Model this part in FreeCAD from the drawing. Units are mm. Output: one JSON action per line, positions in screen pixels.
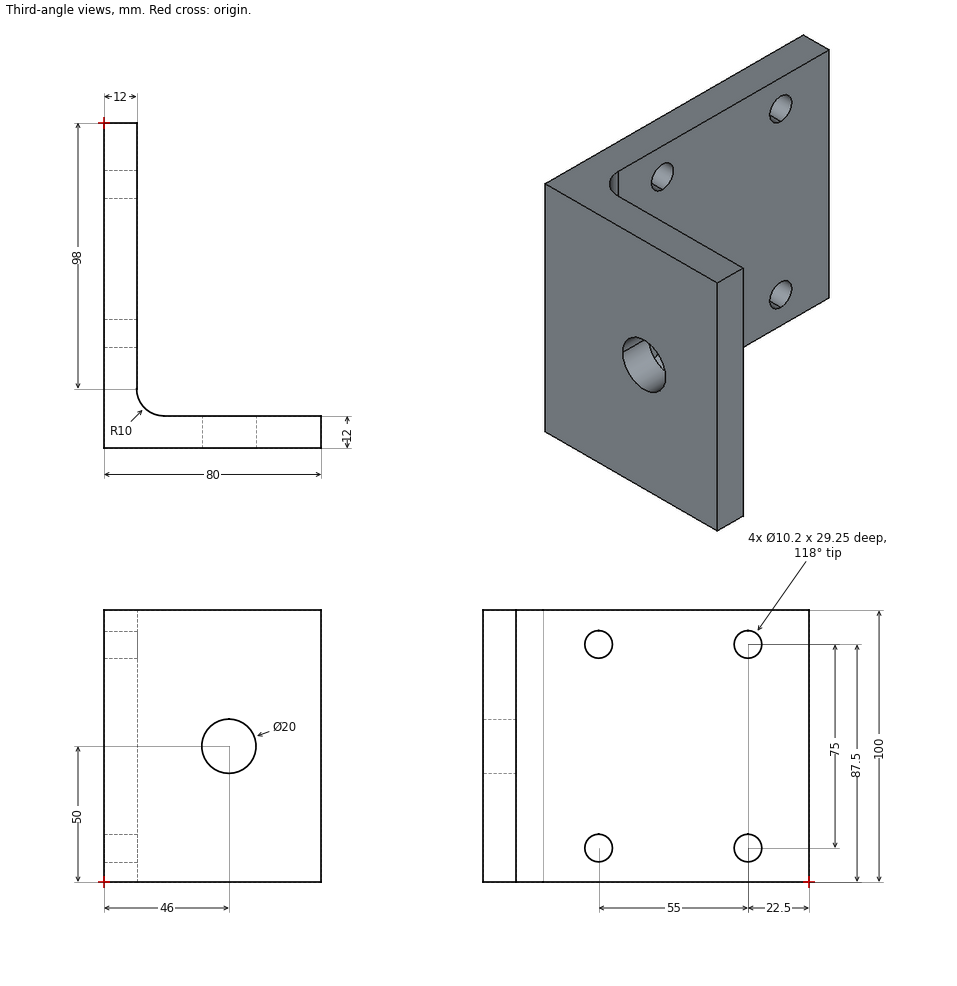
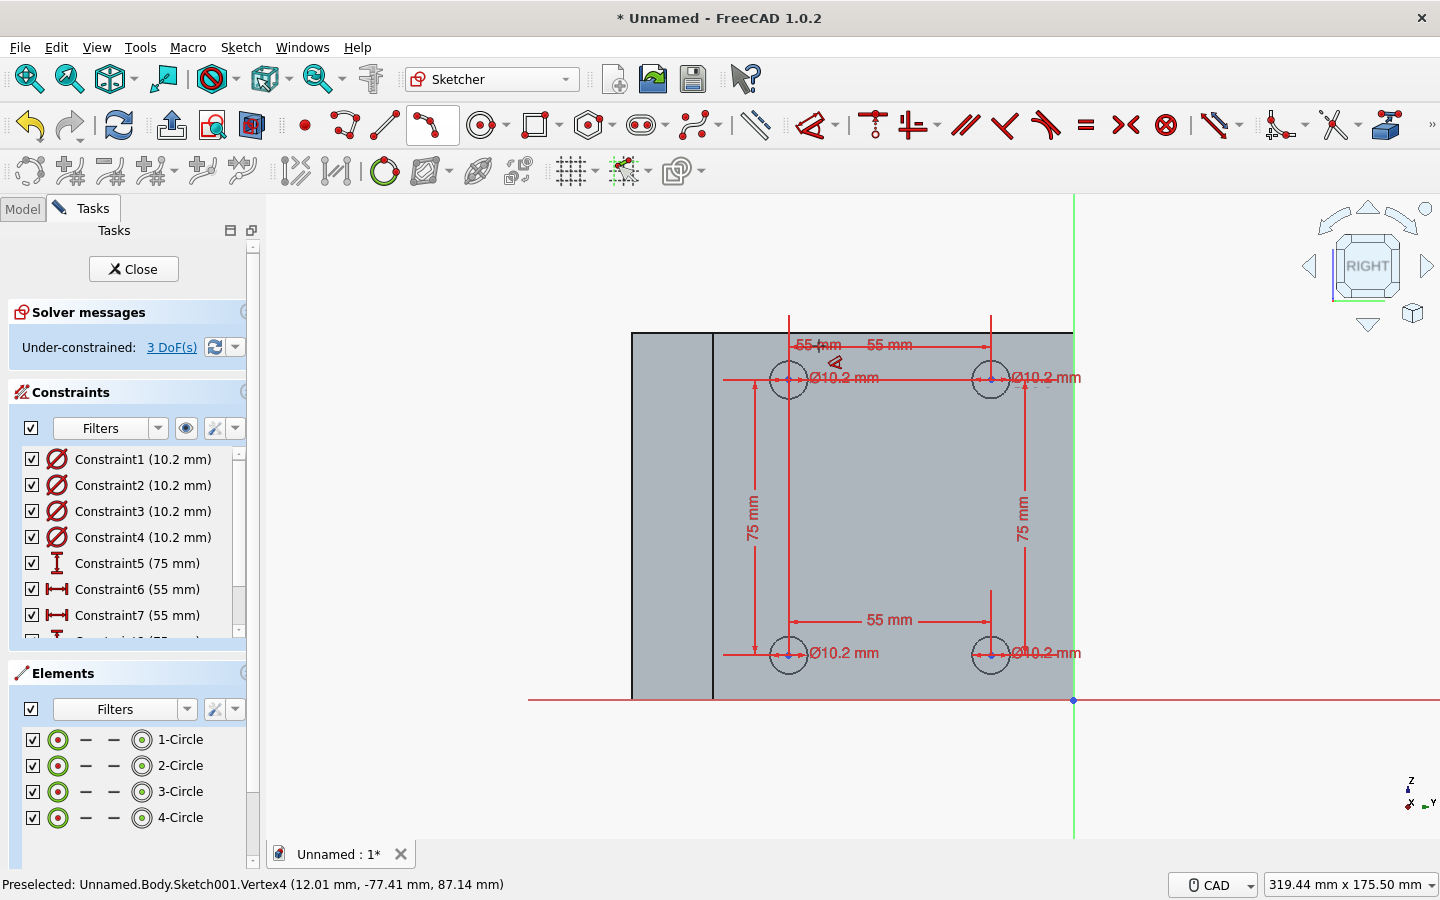
{"action": "left_click", "coordinate": [789, 655]}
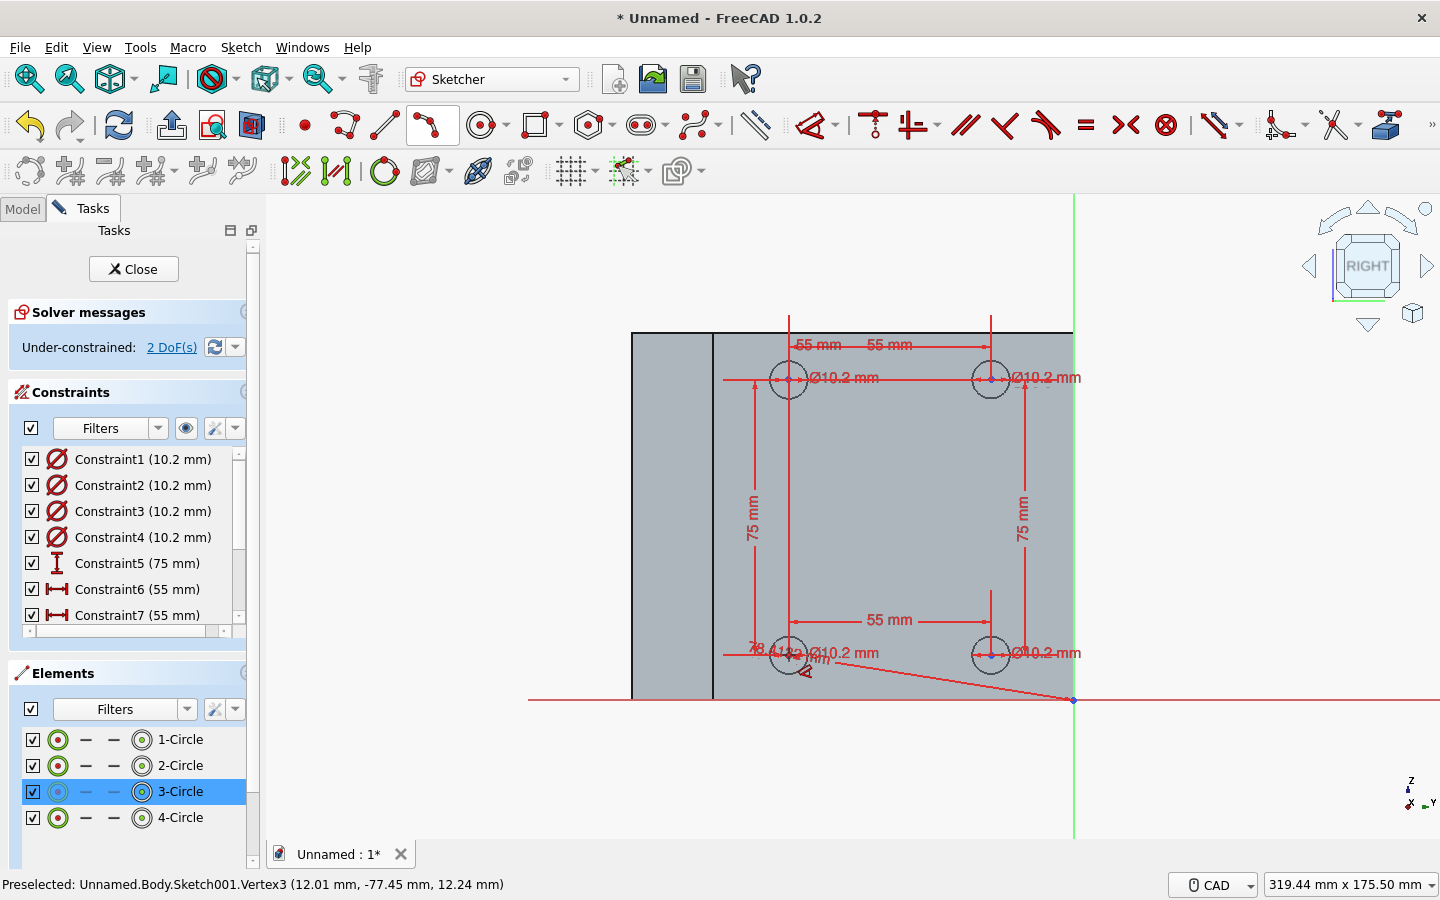
{"action": "left_click", "coordinate": [789, 380]}
{"action": "left_click", "coordinate": [755, 454]}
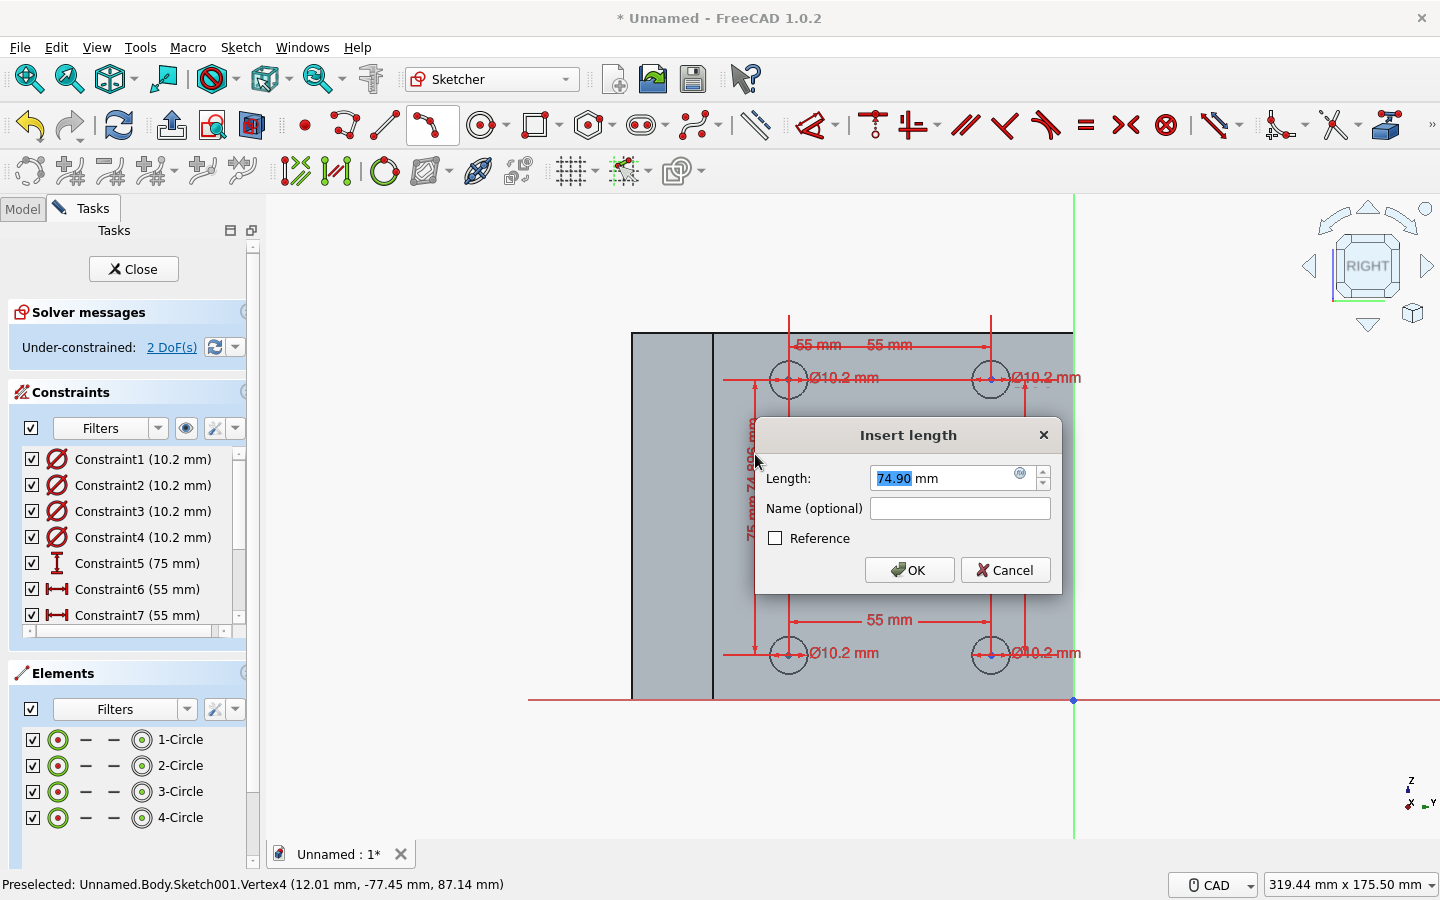
{"action": "type", "text": "75"}
{"action": "key", "text": "Return"}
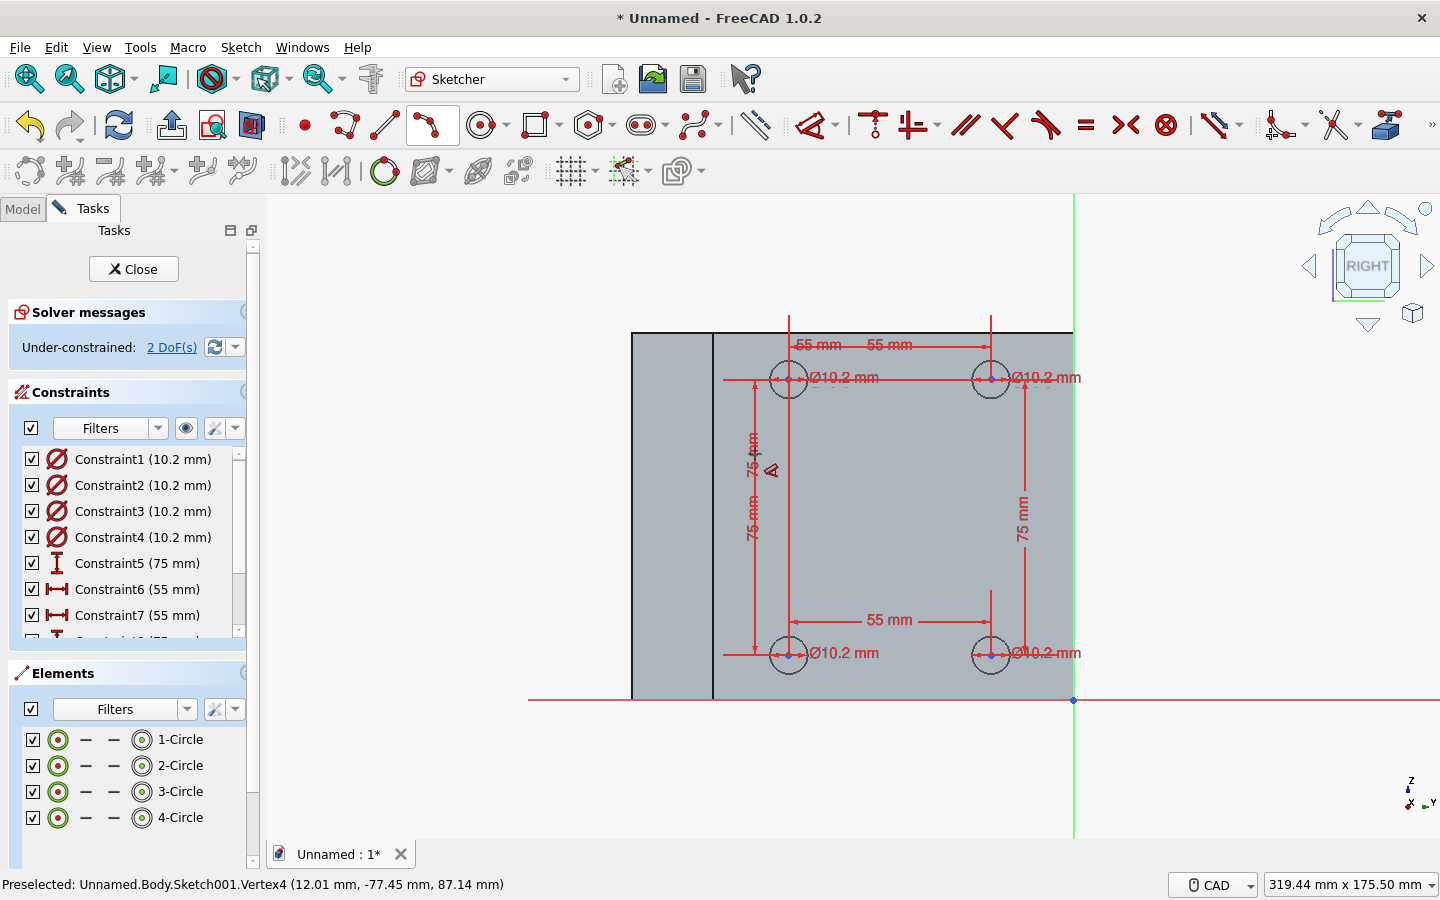
{"action": "left_click", "coordinate": [991, 380]}
{"action": "left_click", "coordinate": [1032, 734]}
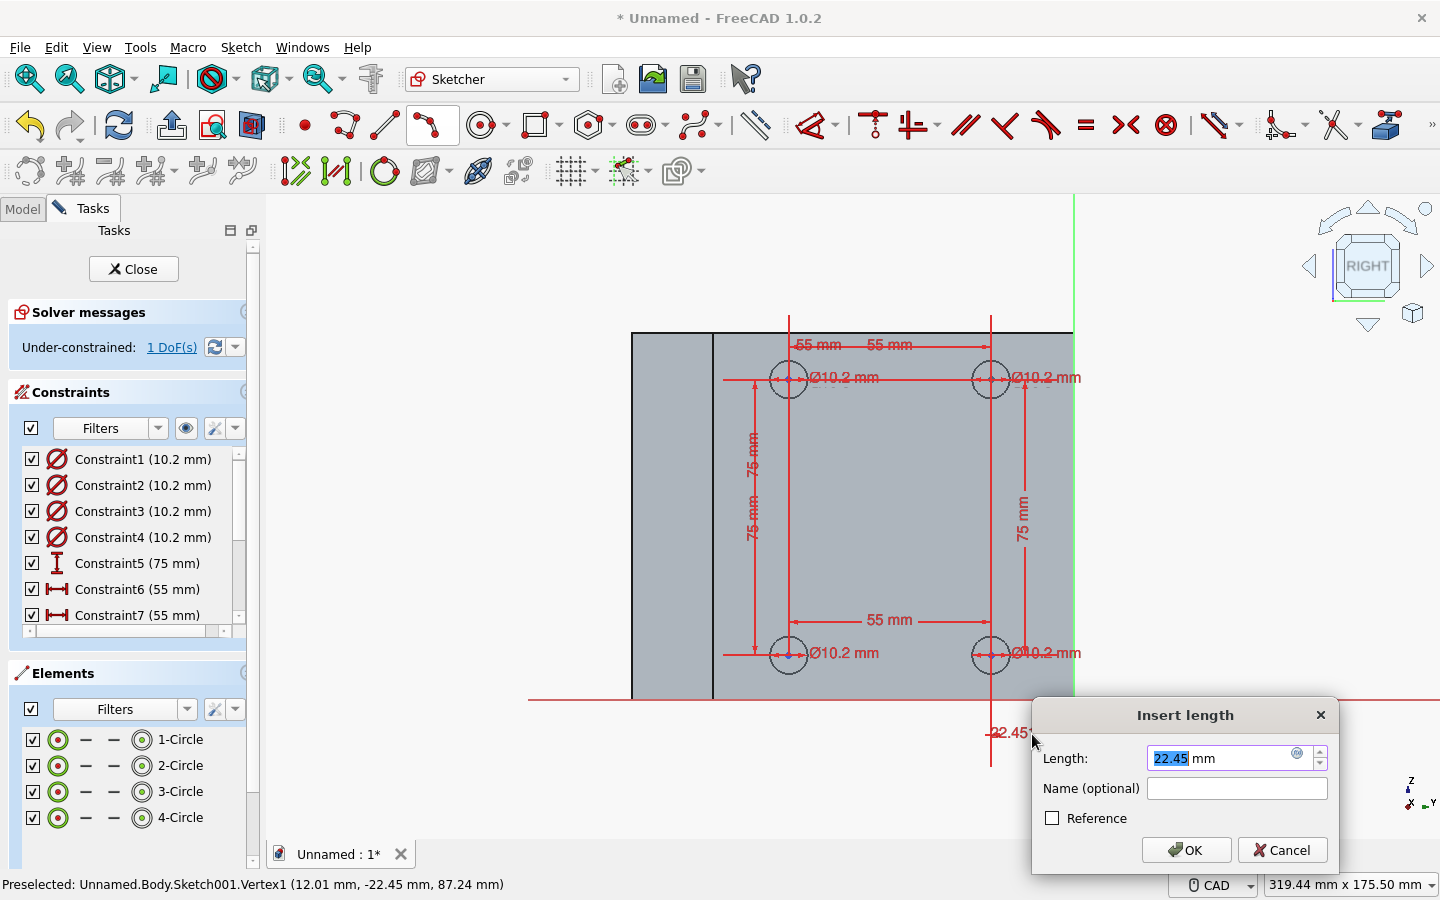
{"action": "type", "text": "22.5"}
{"action": "key", "text": "Return"}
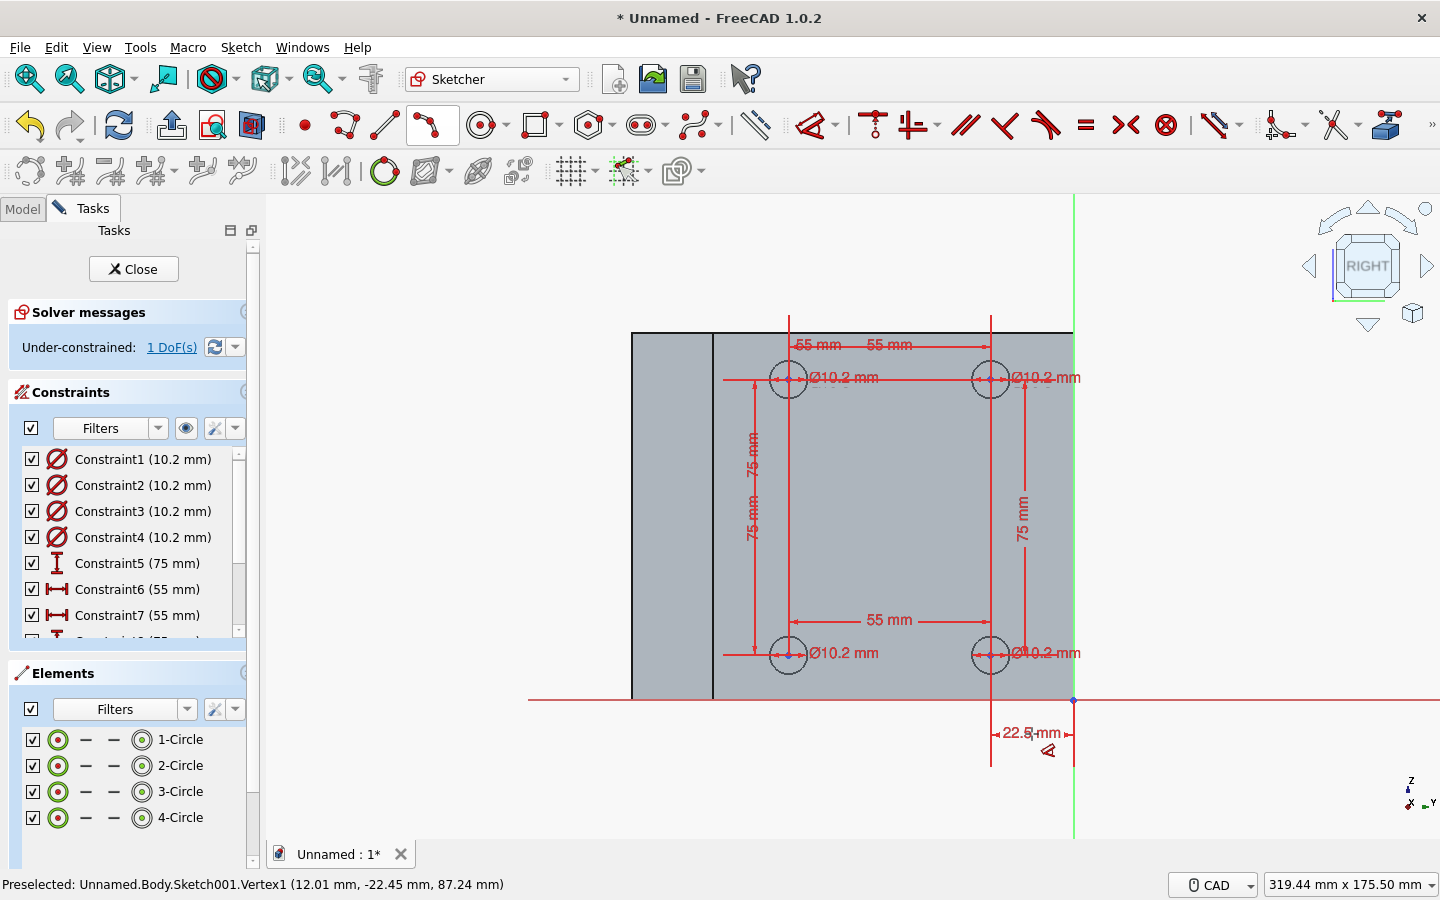
{"action": "left_click", "coordinate": [991, 380]}
{"action": "left_click", "coordinate": [1108, 540]}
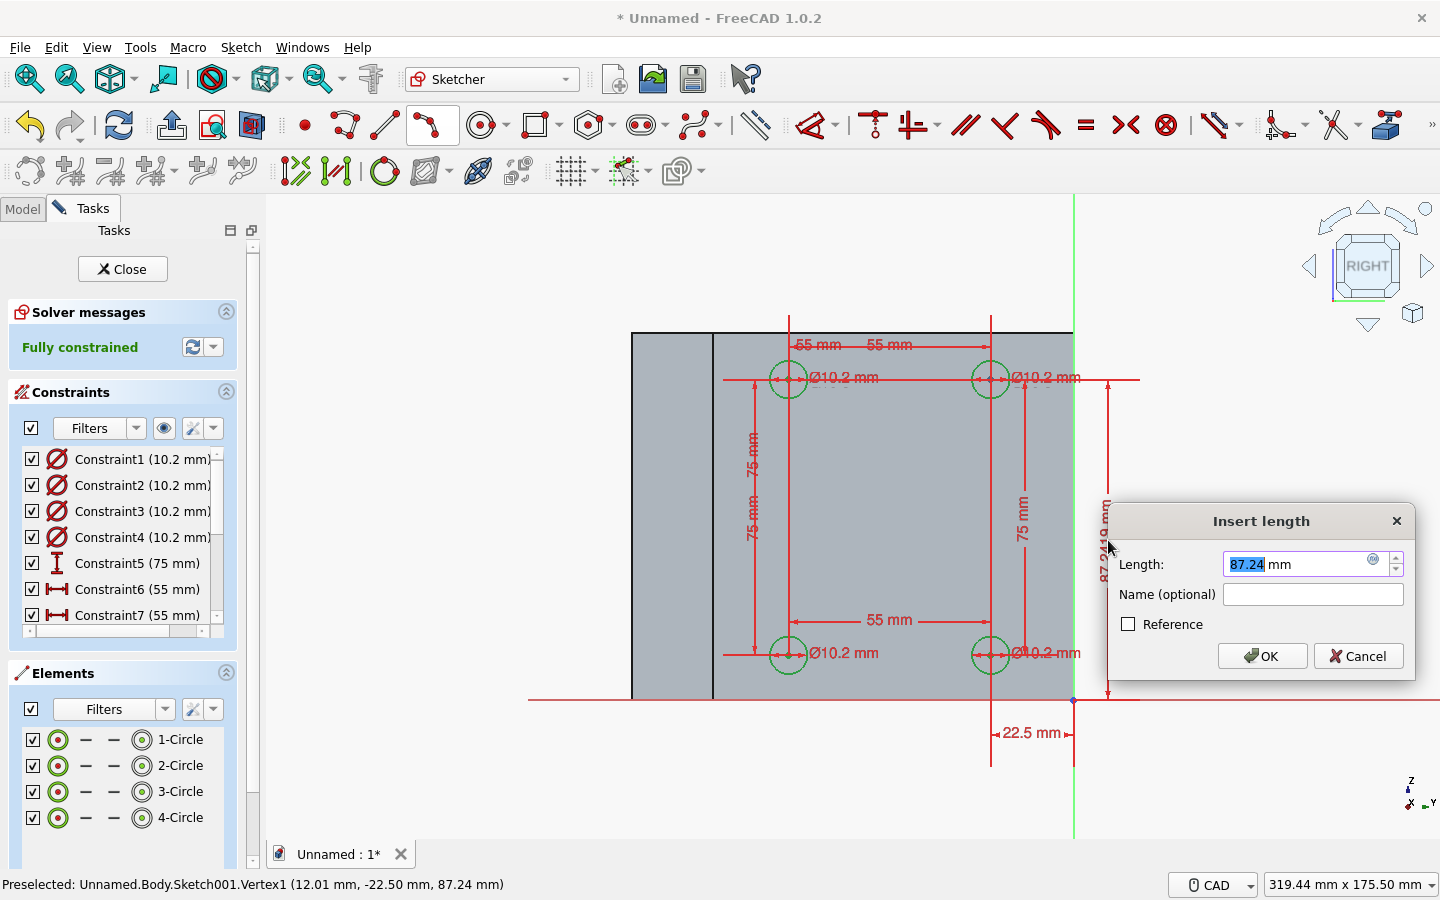
{"action": "type", "text": "87.5"}
{"action": "key", "text": "Return"}
{"action": "key", "text": "Escape"}